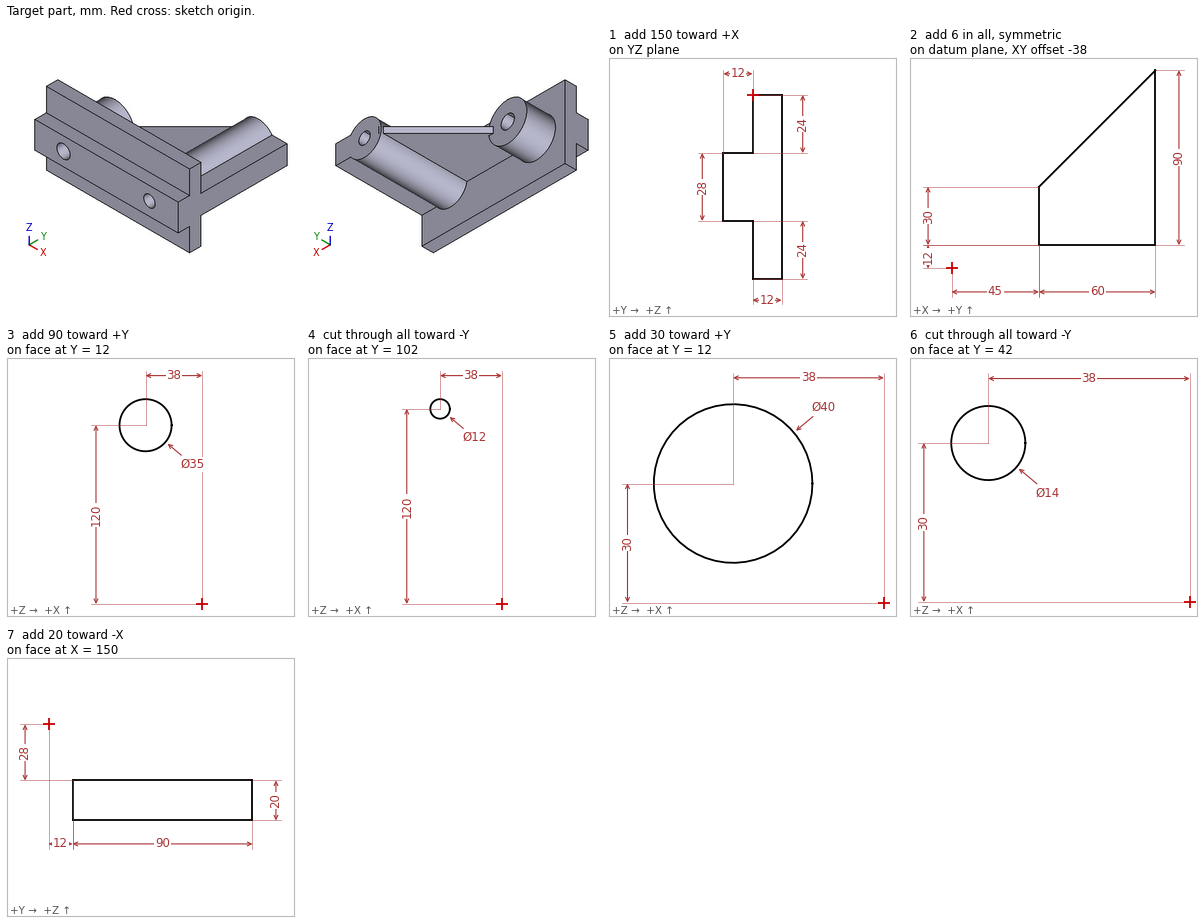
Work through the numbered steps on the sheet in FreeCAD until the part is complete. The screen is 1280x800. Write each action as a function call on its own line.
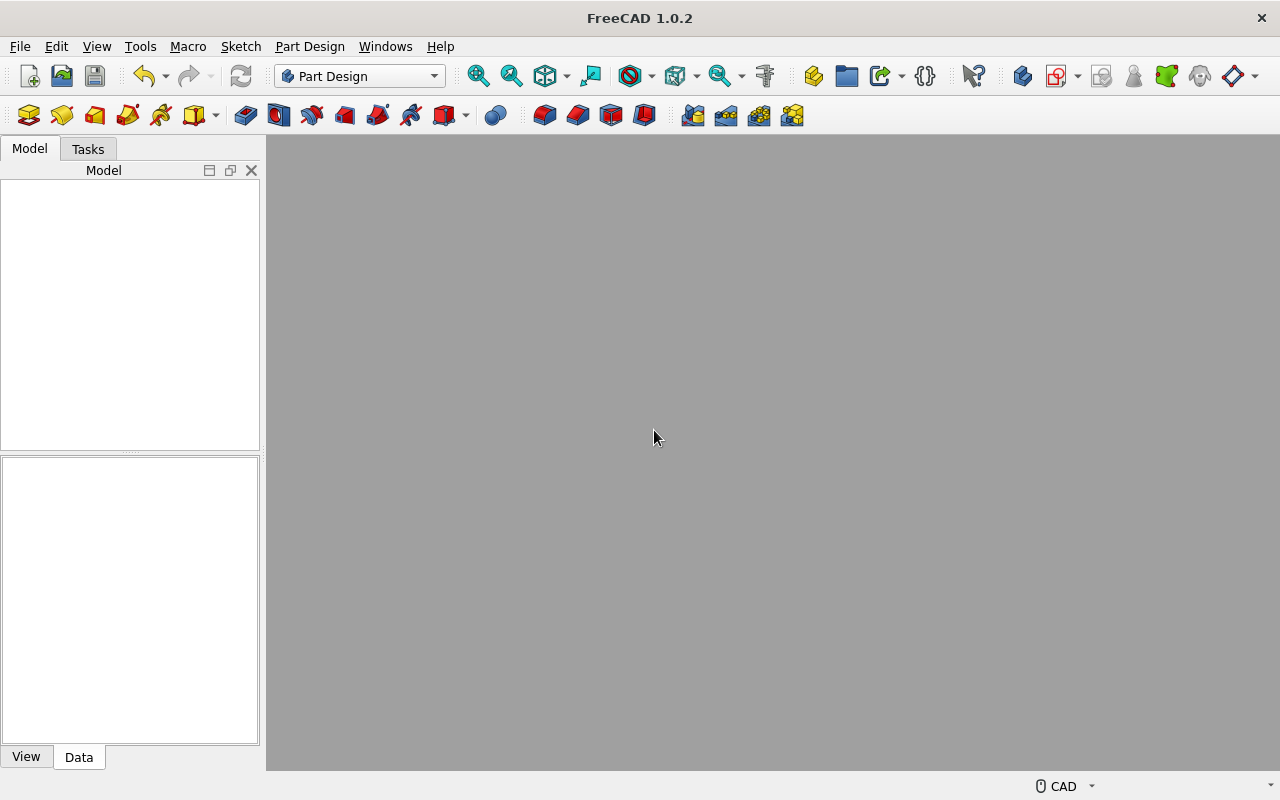
click(29, 76)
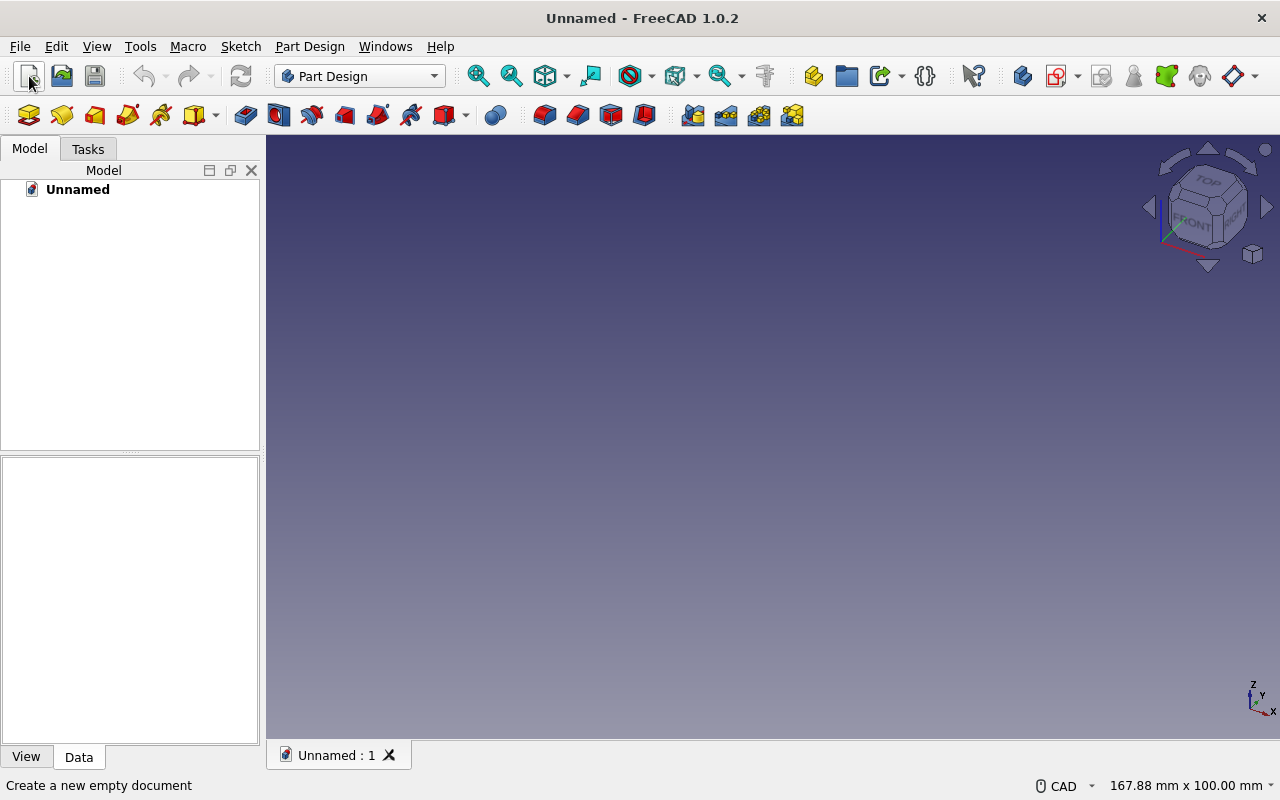
click(1056, 76)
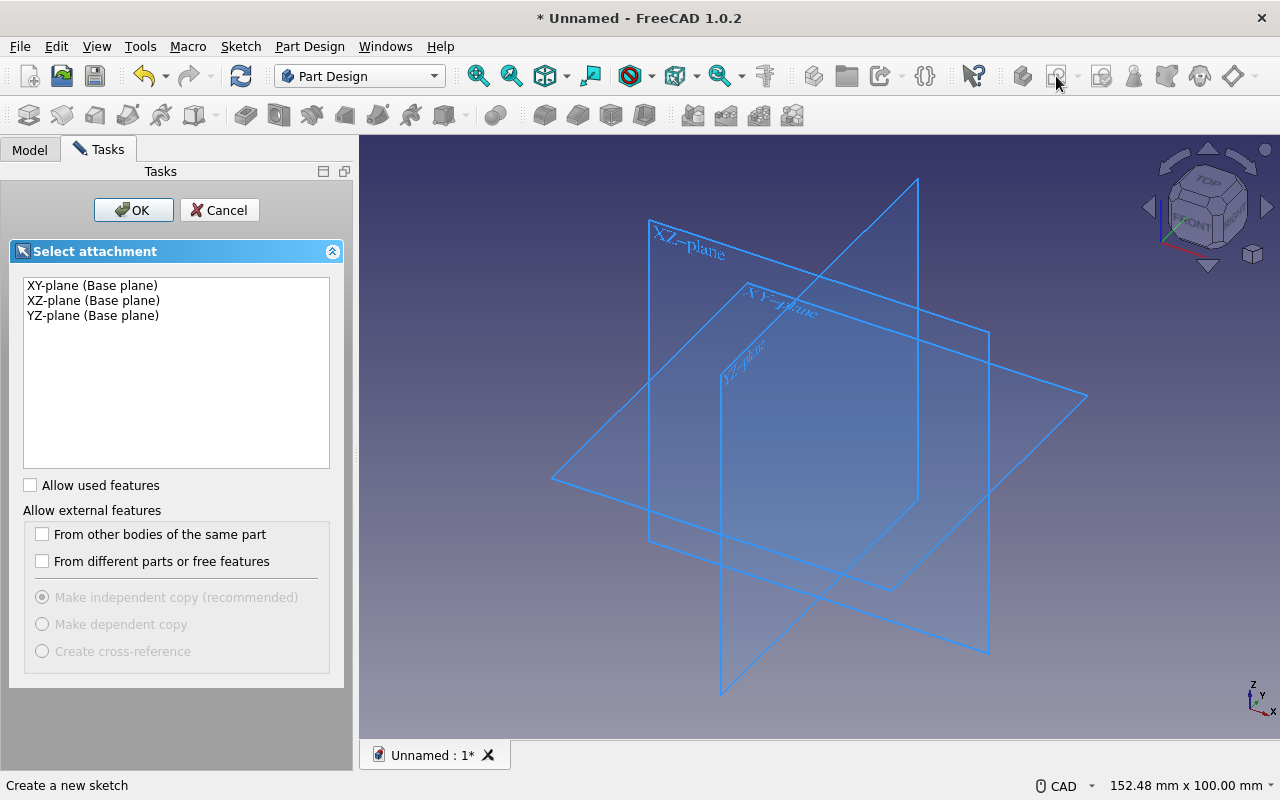
click(84, 316)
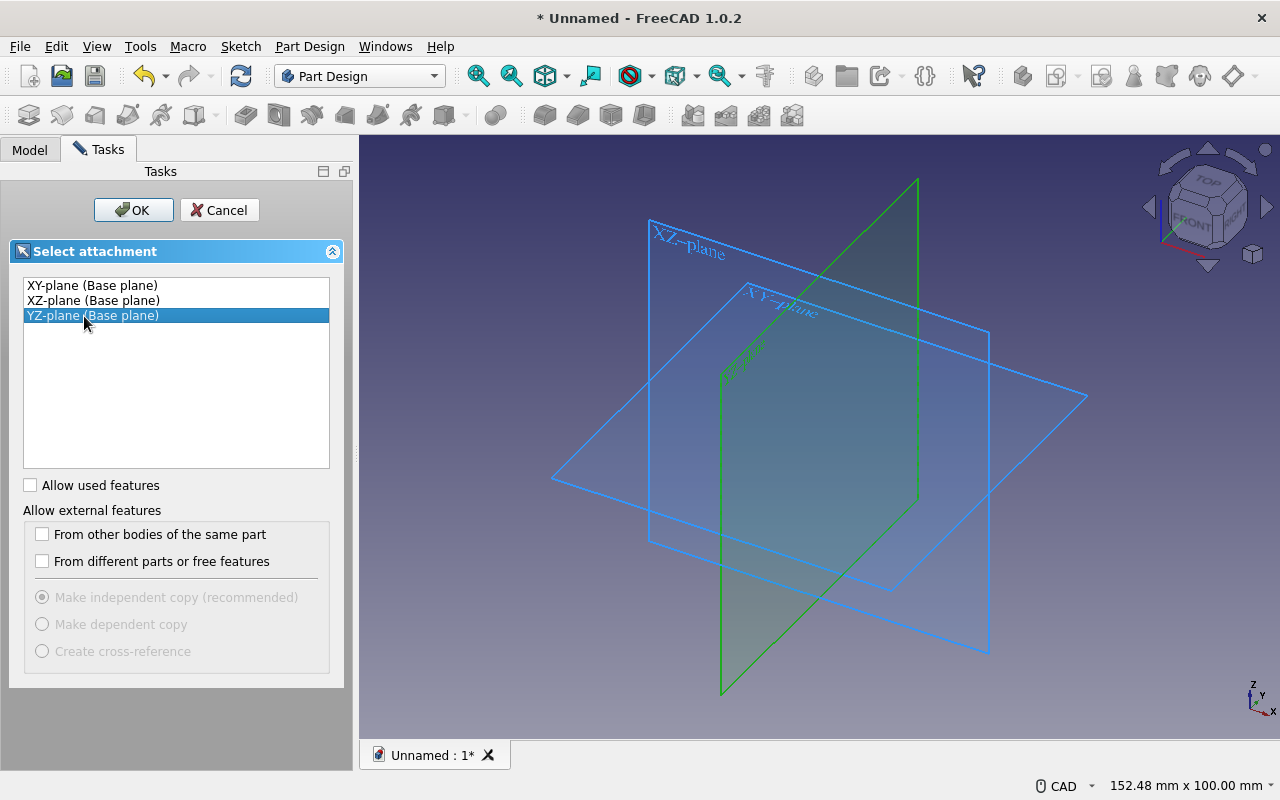
click(134, 210)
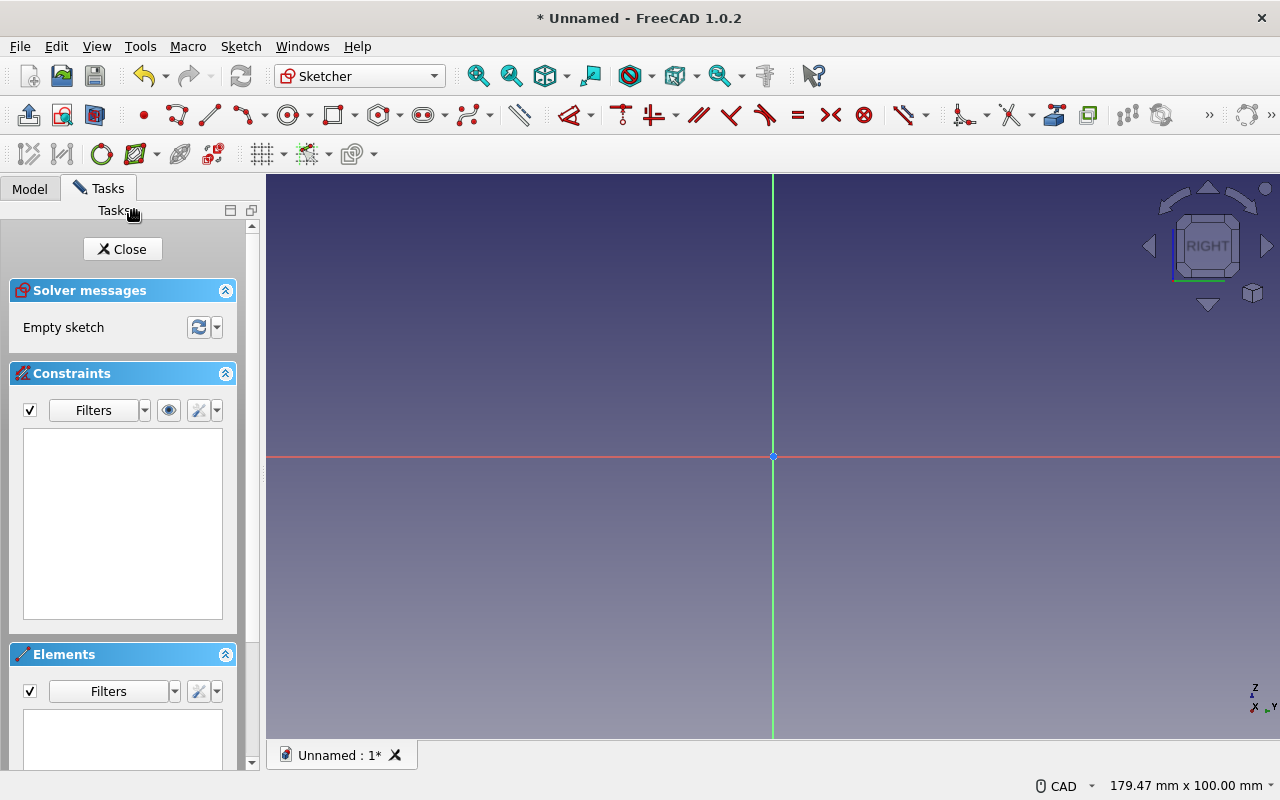
scroll(565, 202, down, 2)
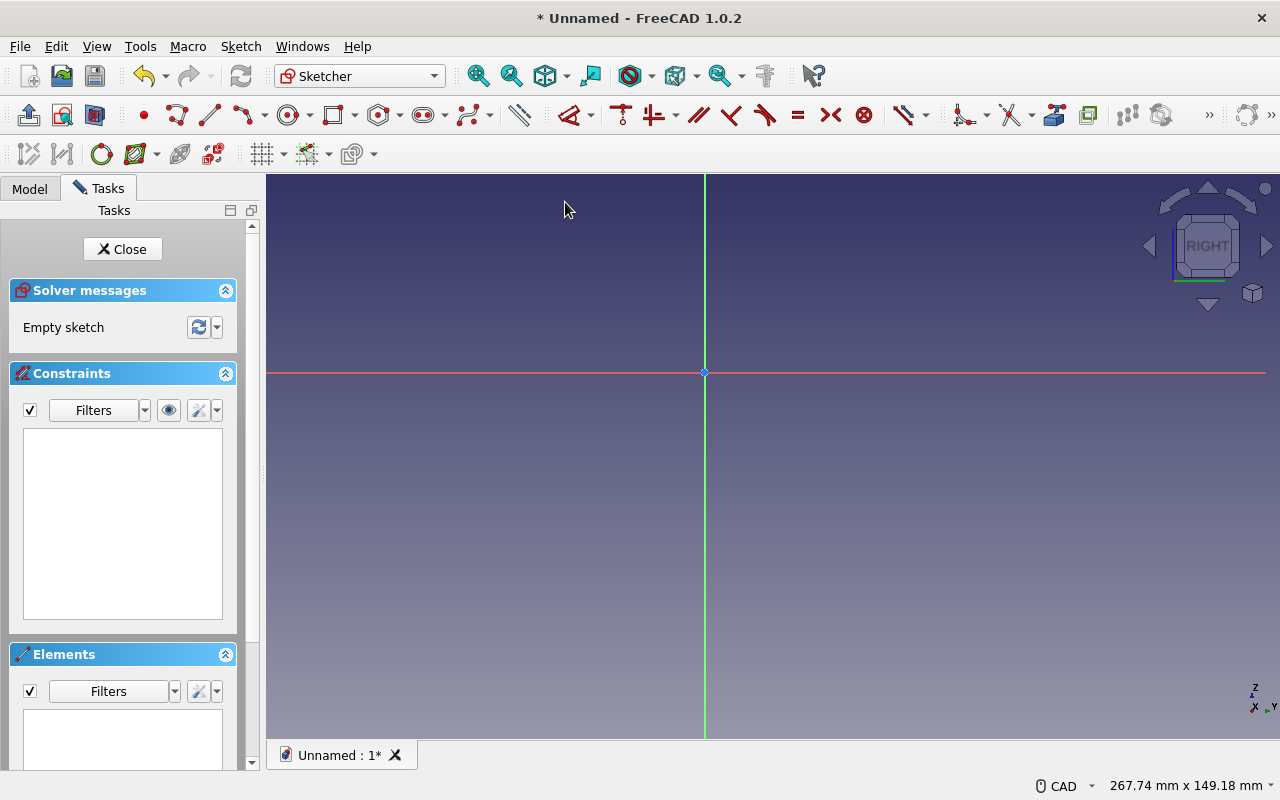
click(177, 116)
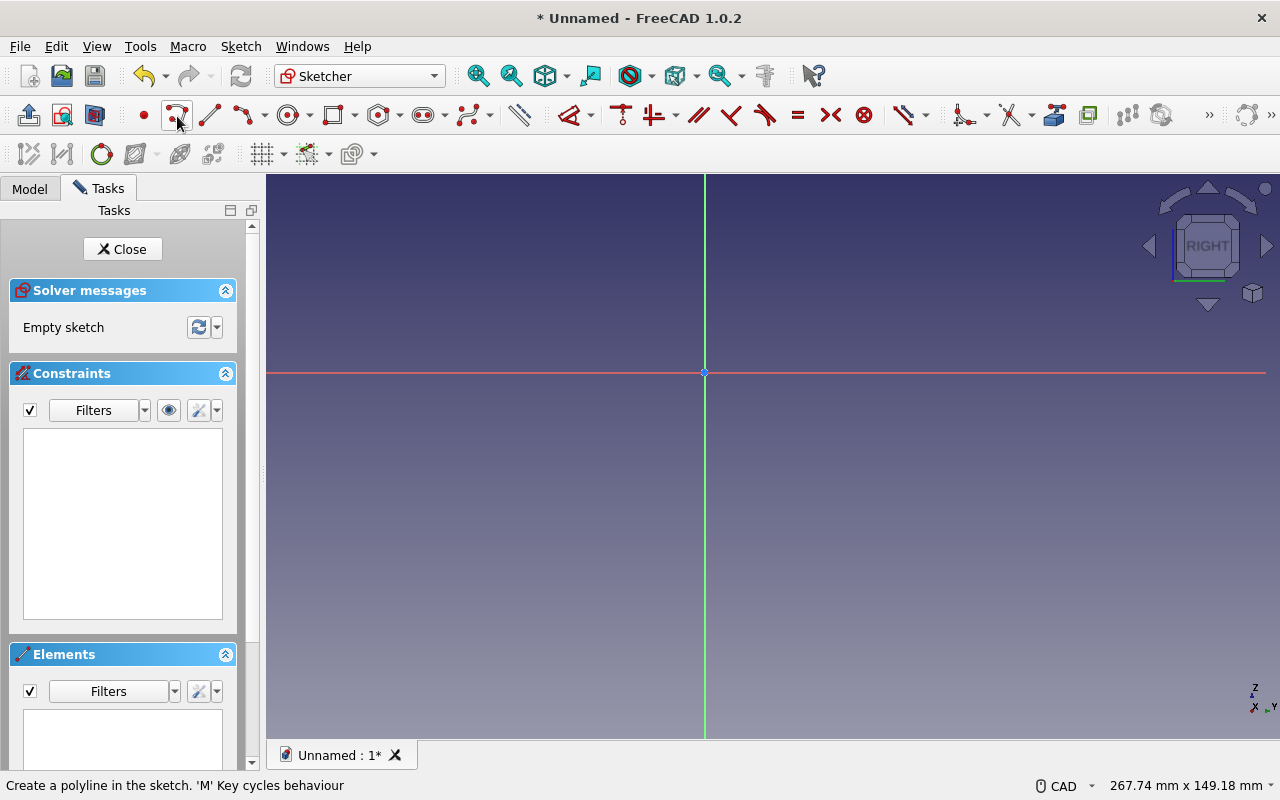
click(705, 373)
click(714, 464)
click(659, 464)
click(659, 570)
click(705, 570)
click(714, 660)
click(750, 660)
click(750, 382)
click(705, 373)
key(Escape)
key(Escape)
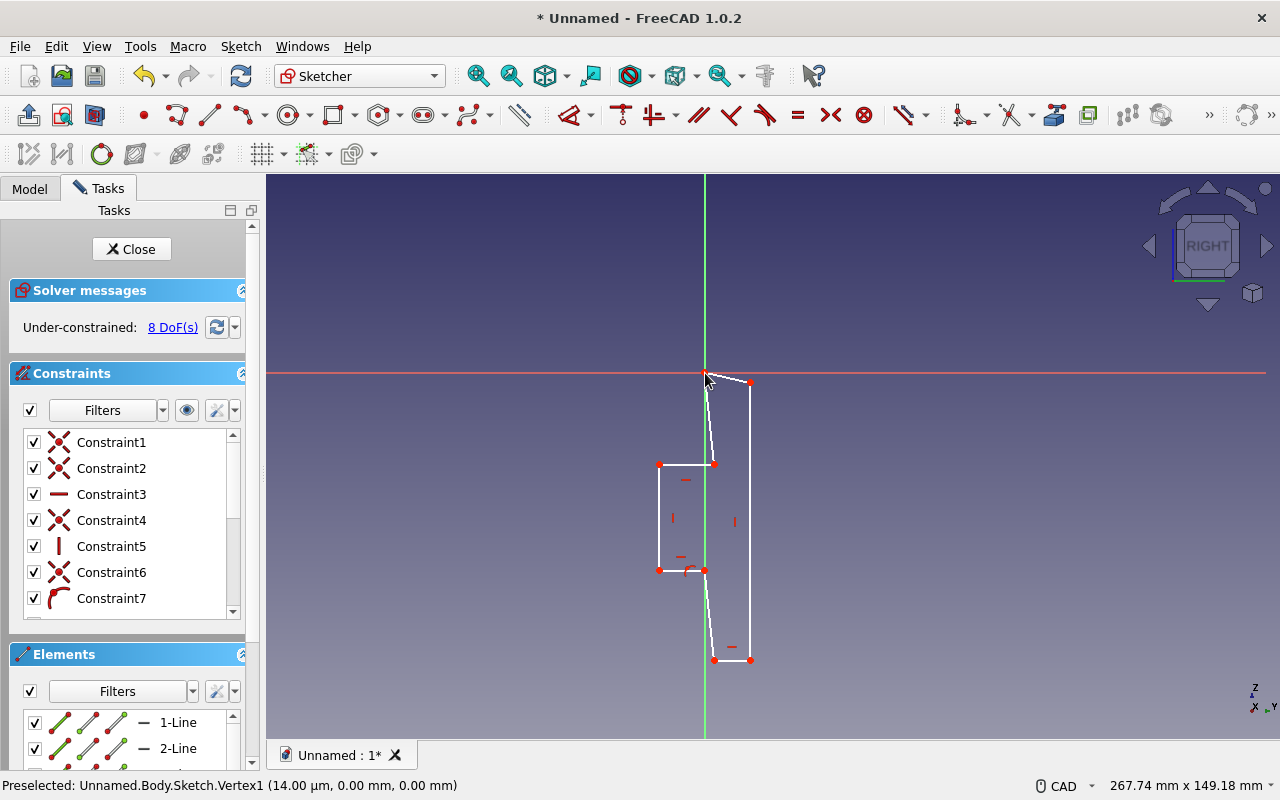
click(707, 400)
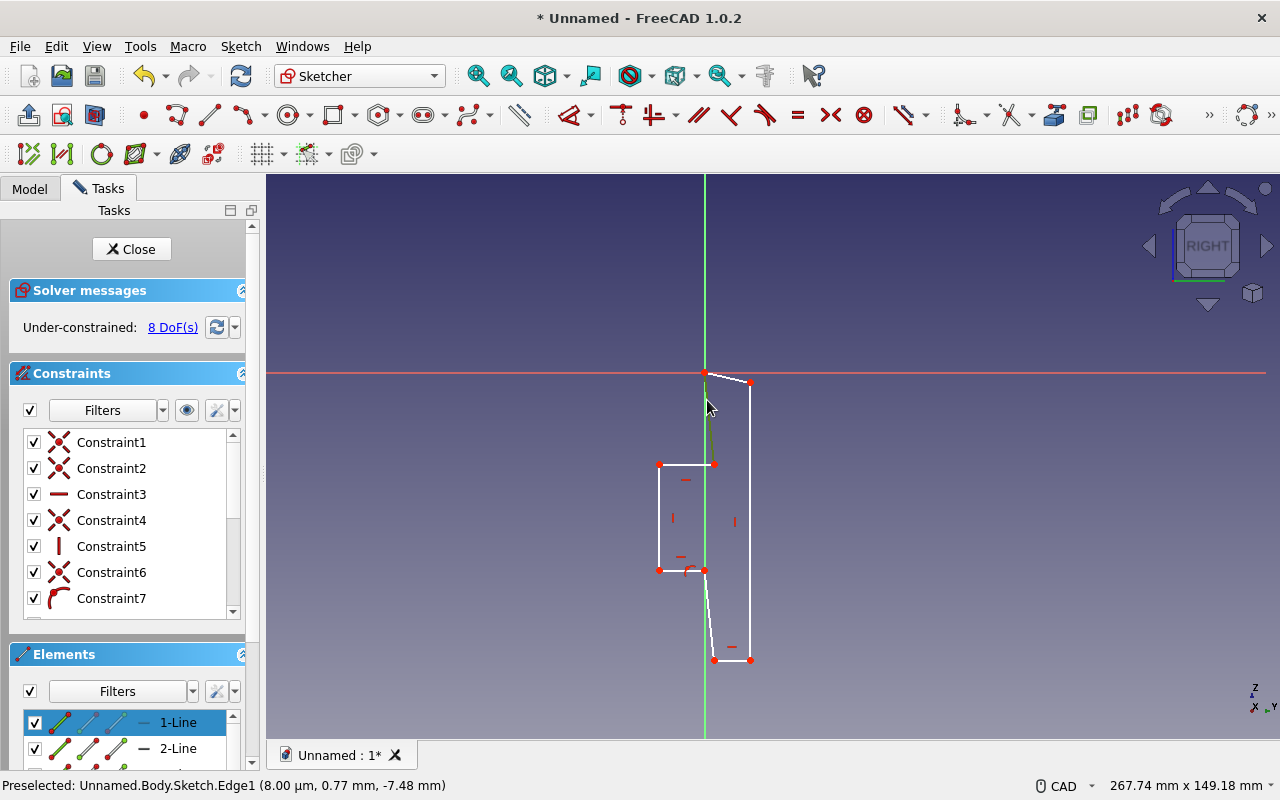
click(676, 116)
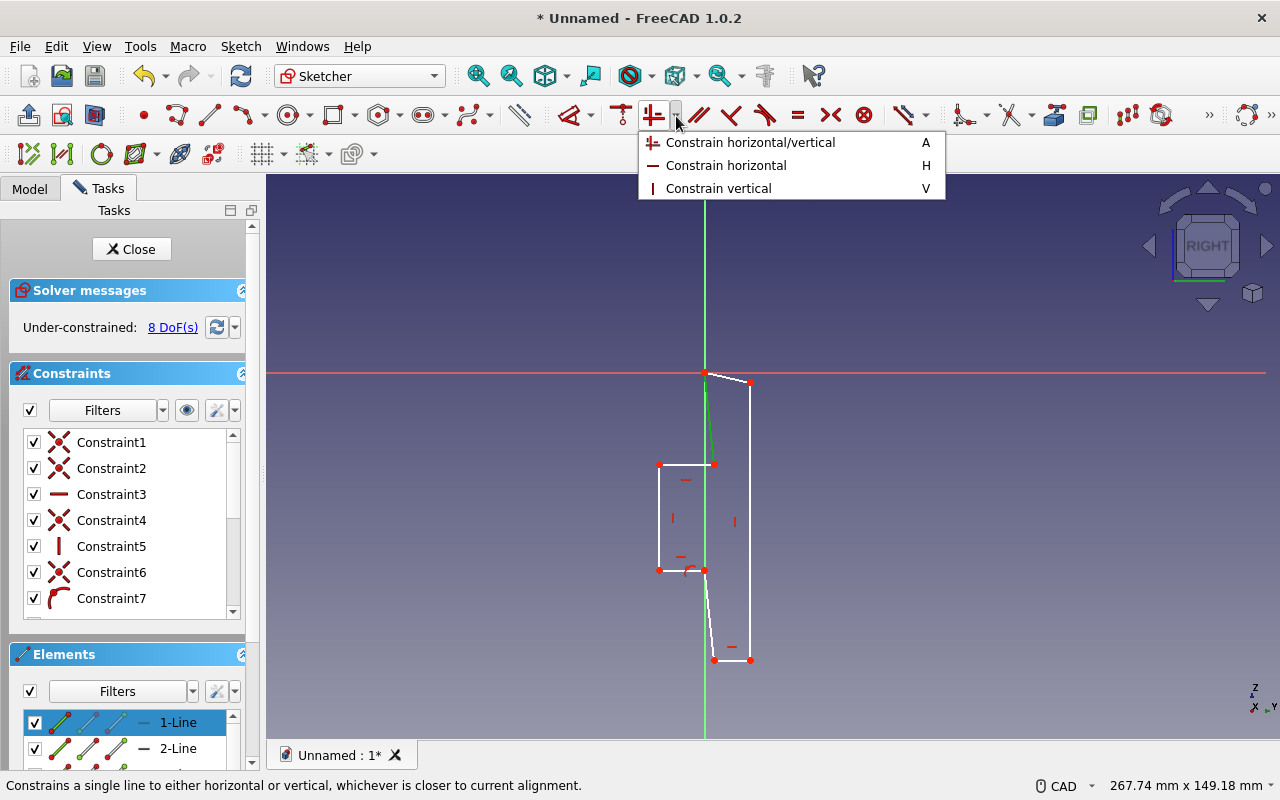
click(792, 188)